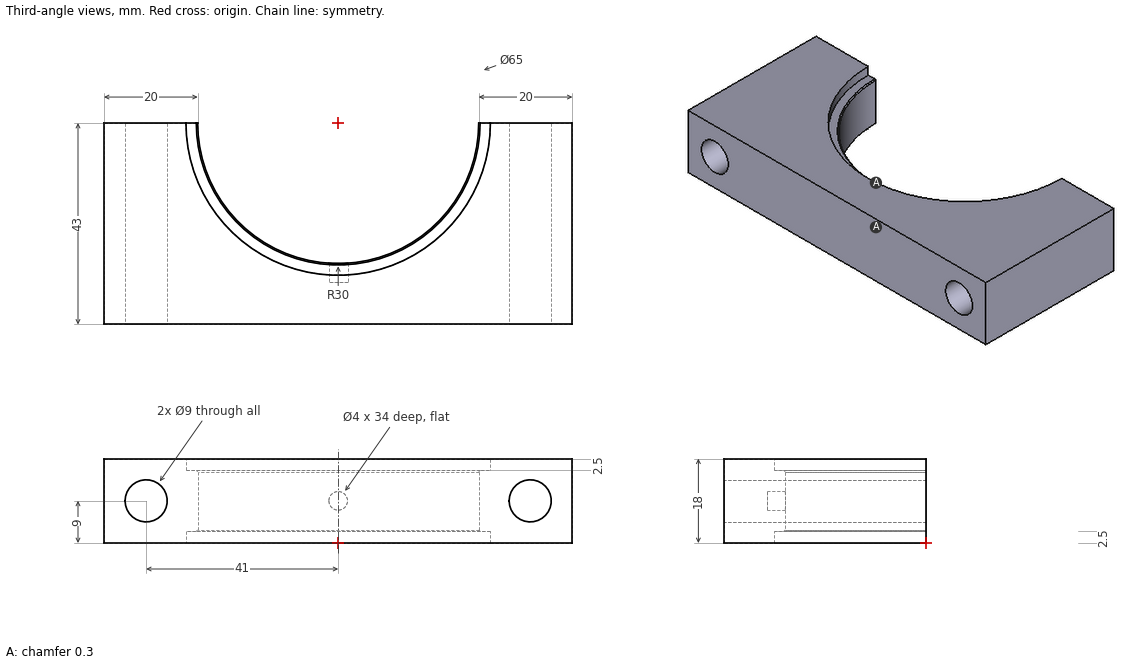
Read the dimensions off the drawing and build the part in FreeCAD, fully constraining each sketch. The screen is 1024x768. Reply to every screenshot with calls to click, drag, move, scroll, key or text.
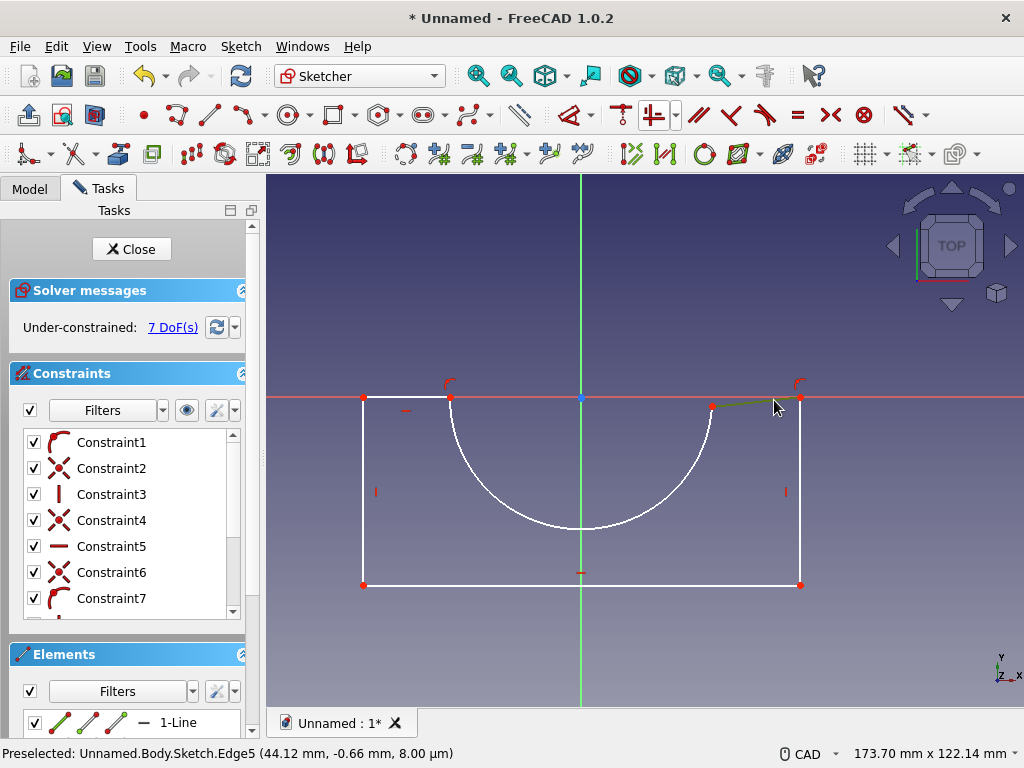
click(676, 116)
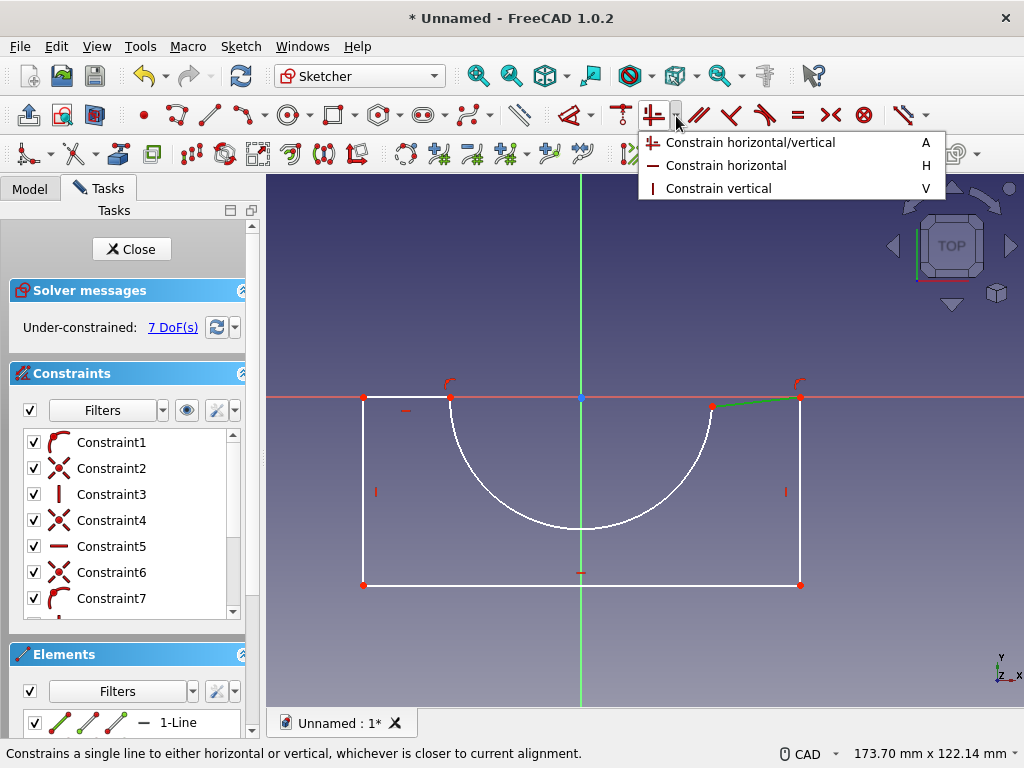
click(792, 166)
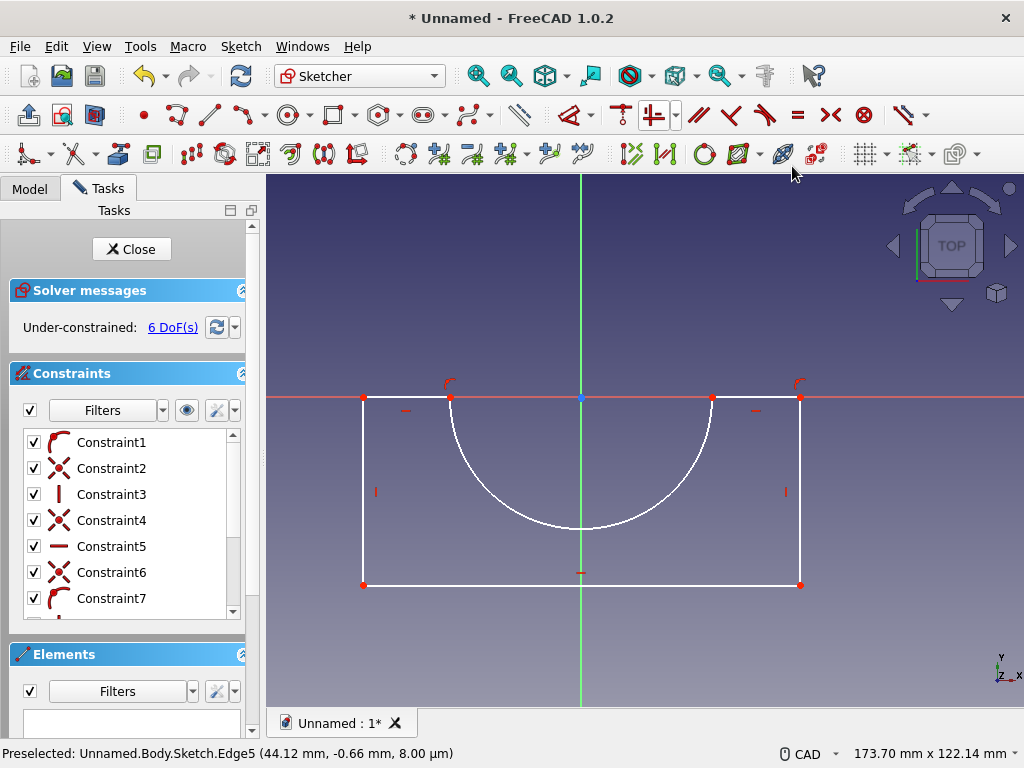
drag(571, 387, 591, 408)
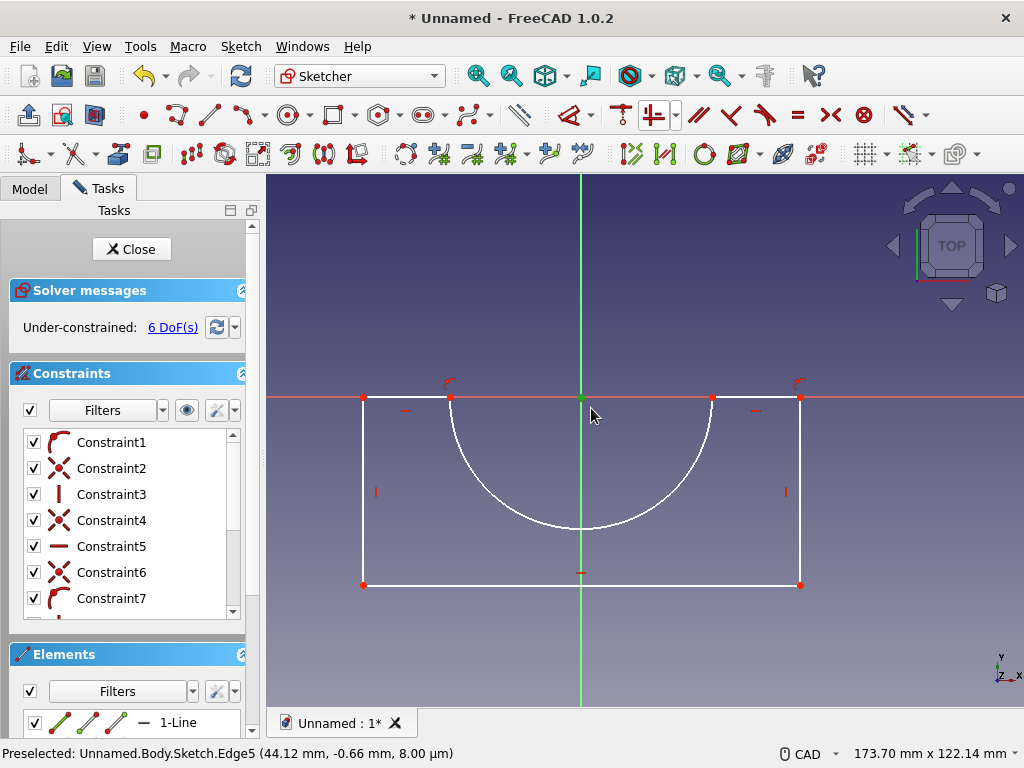
click(621, 116)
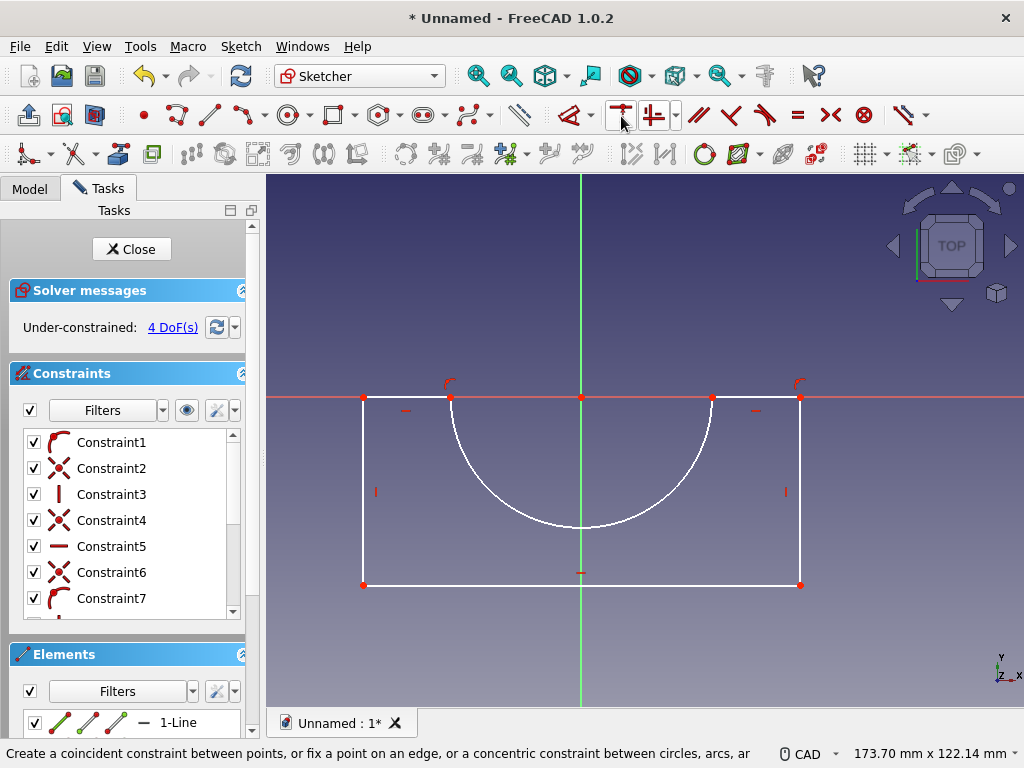
click(568, 116)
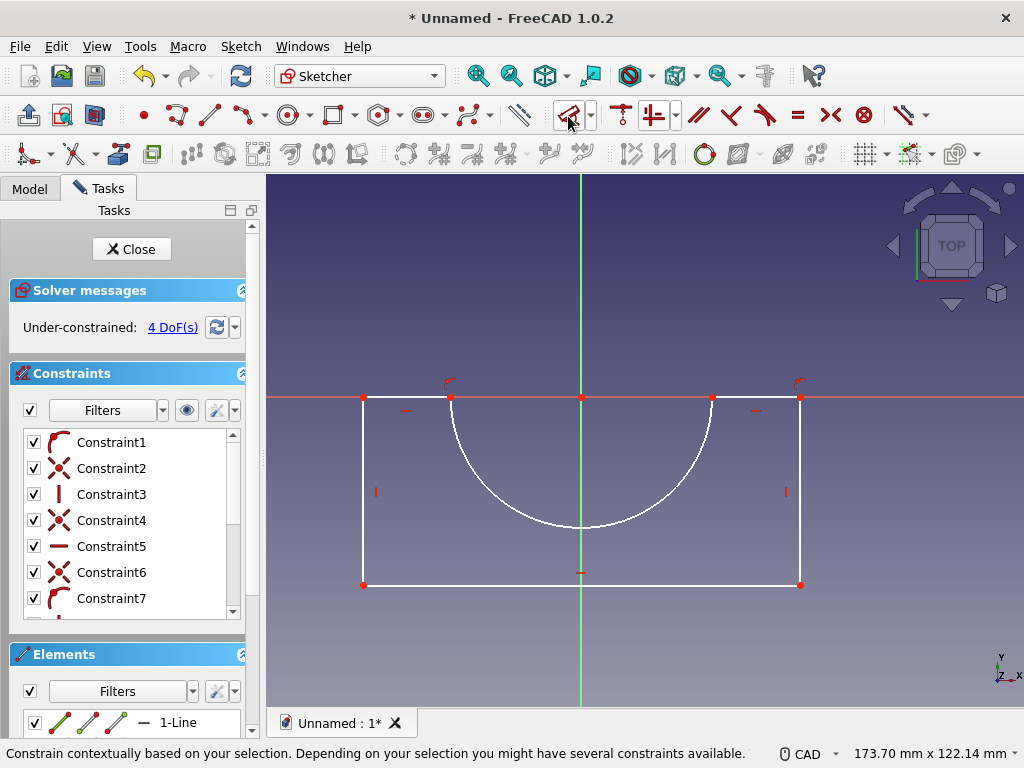
click(505, 503)
click(486, 529)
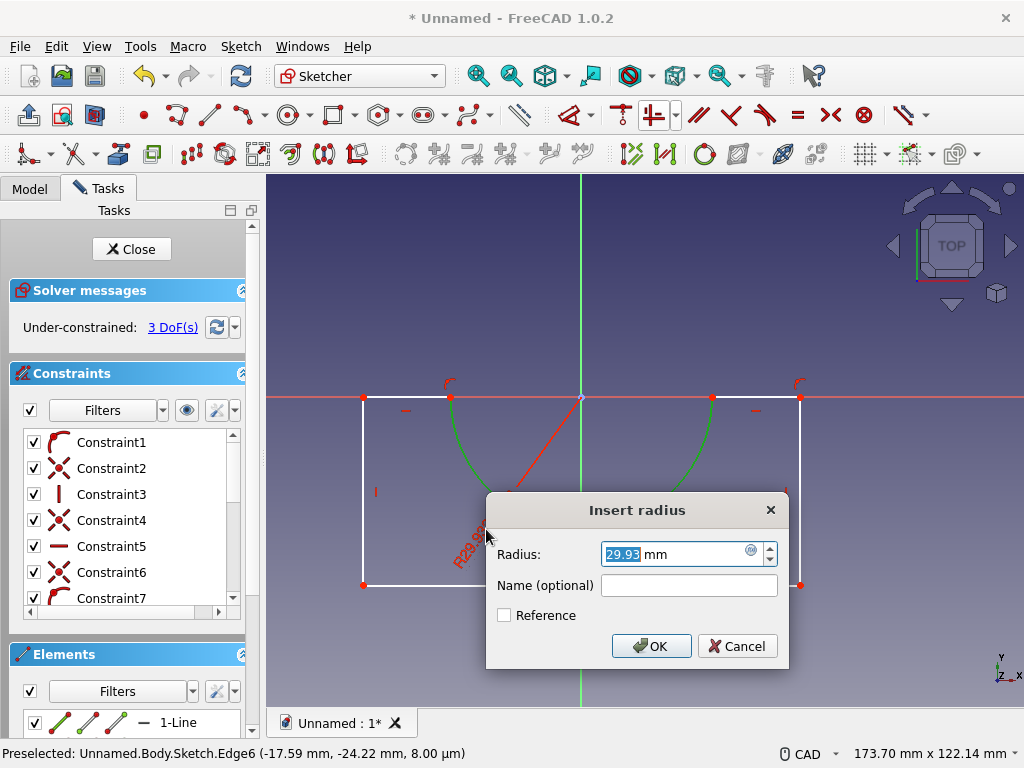
text(30)
key(Return)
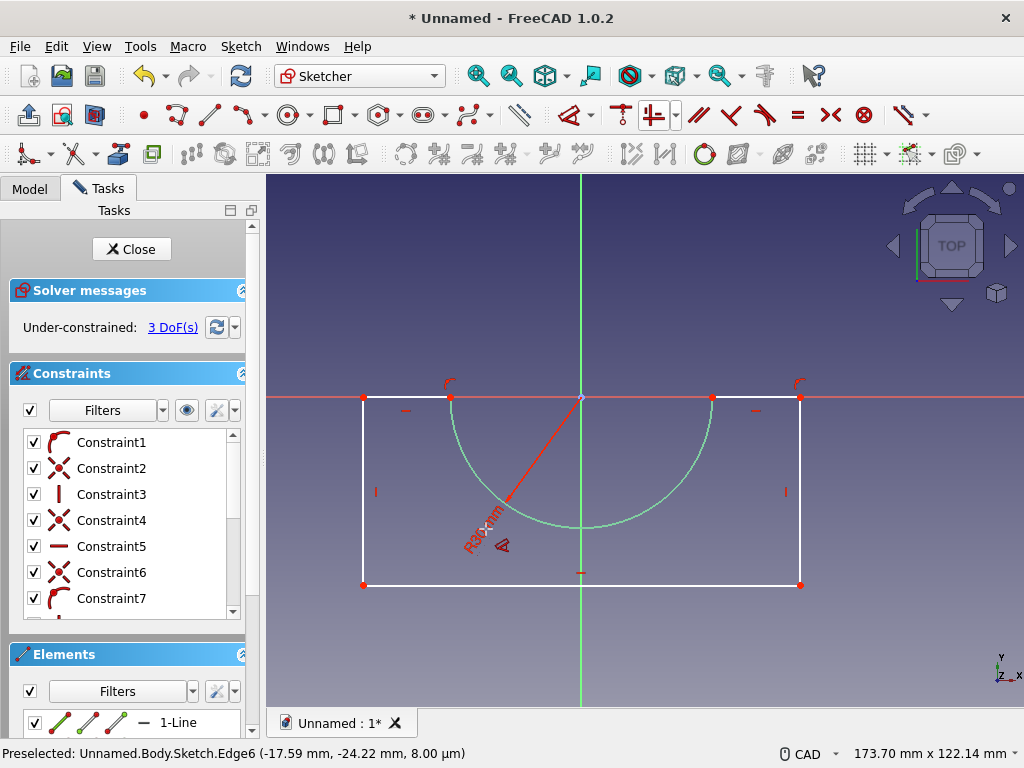
click(424, 397)
click(407, 363)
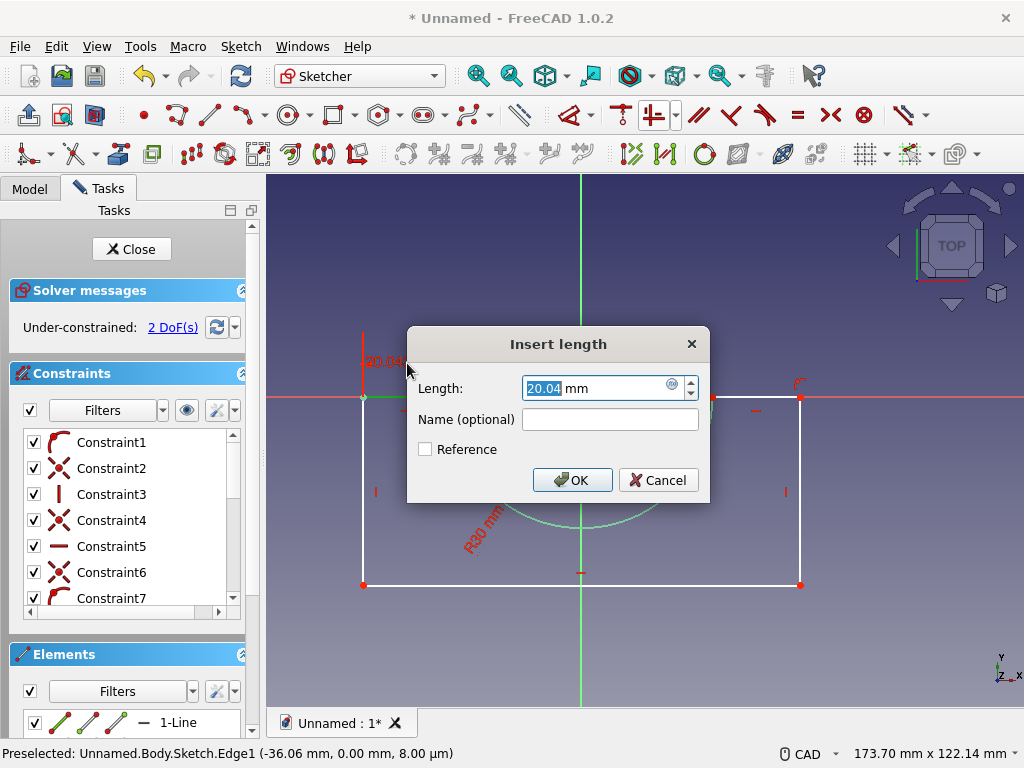
text(20)
key(Return)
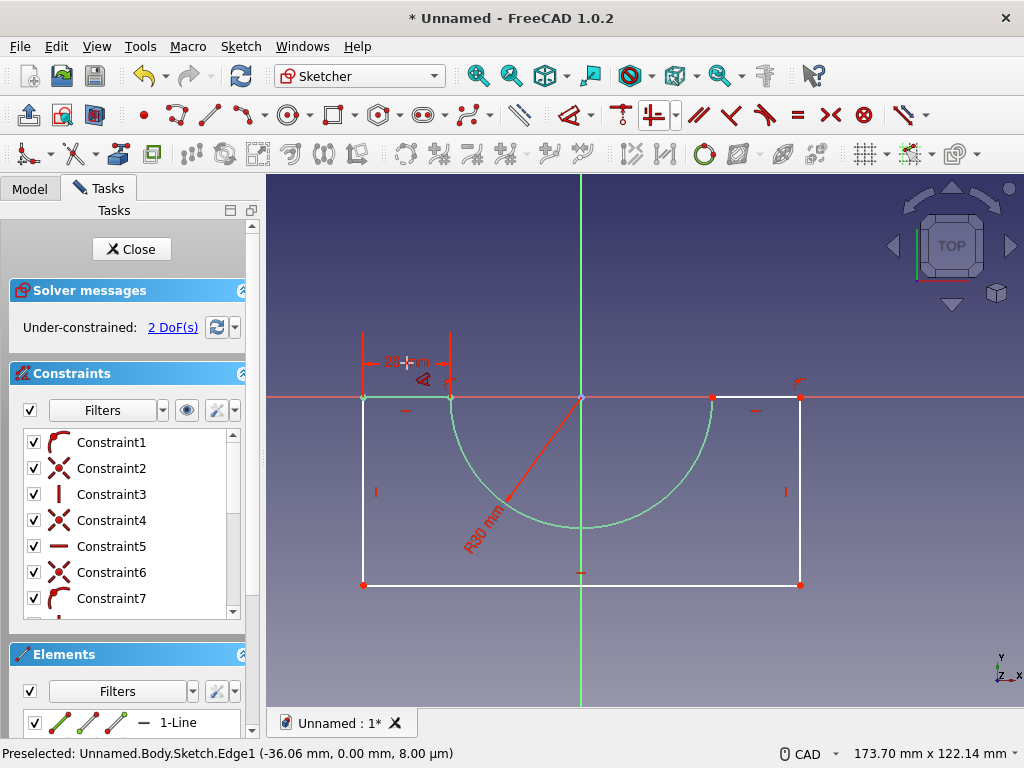
click(363, 454)
click(329, 492)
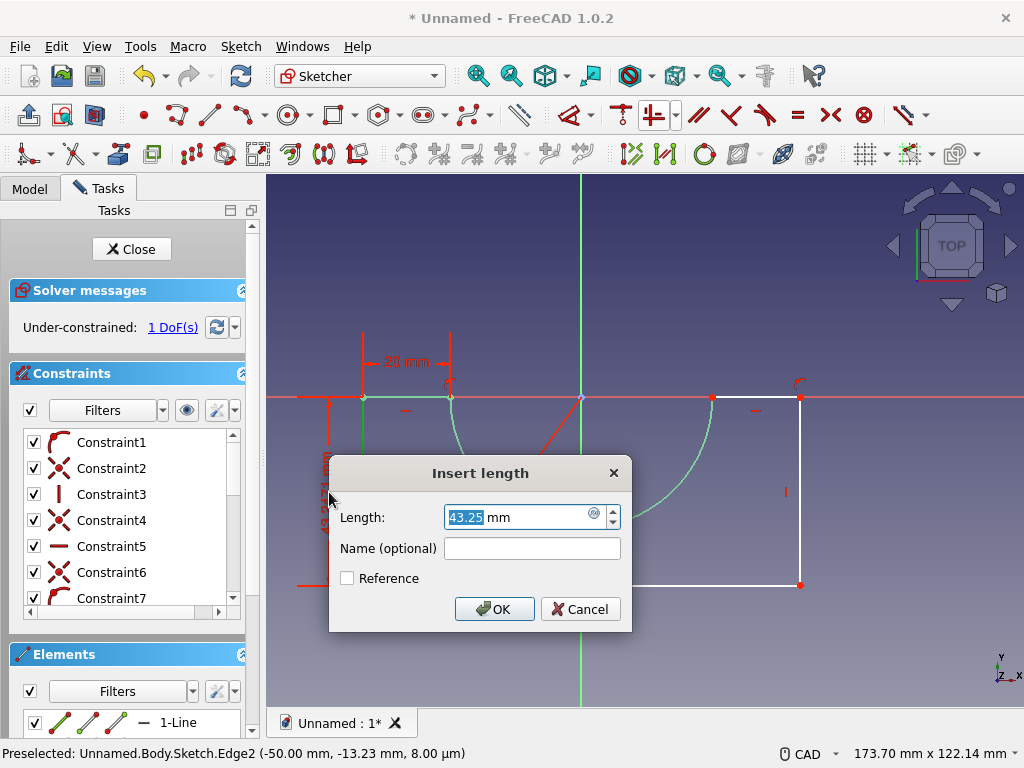
text(43)
key(Return)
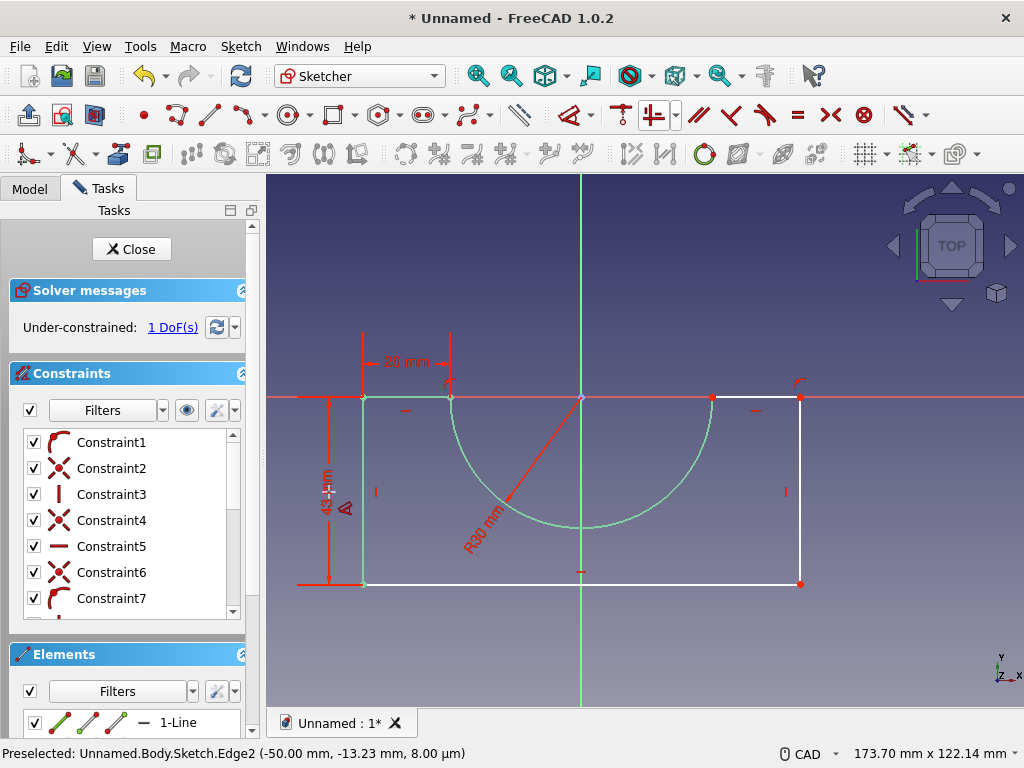
click(774, 397)
click(756, 363)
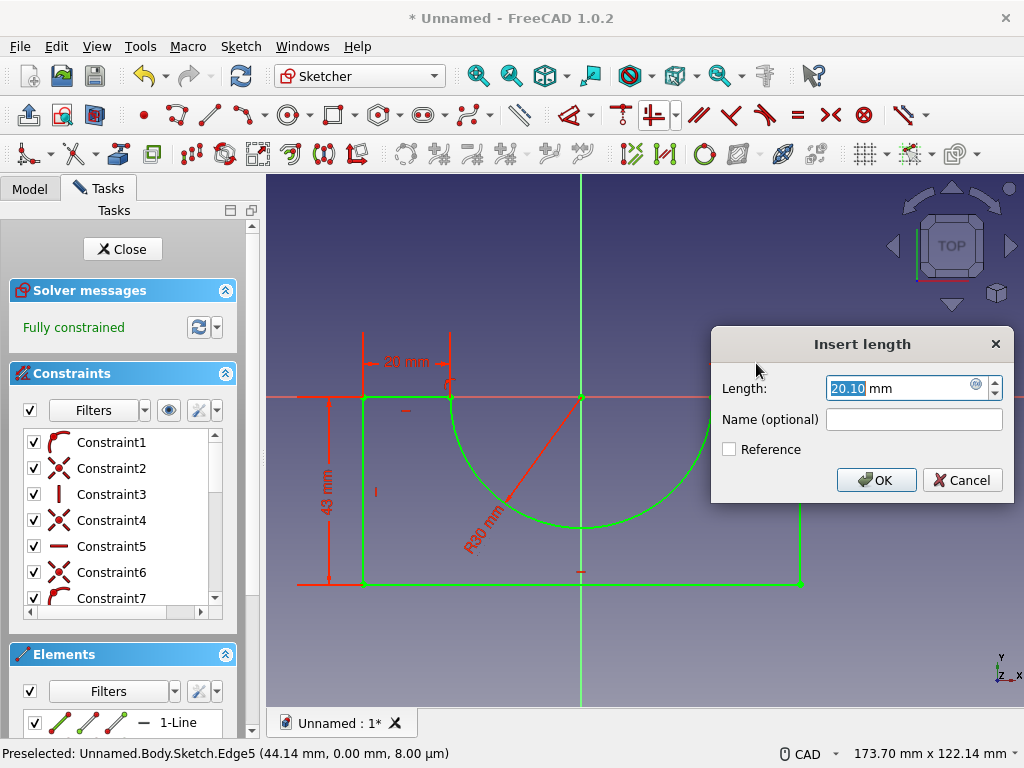
text(20)
key(Return)
key(Escape)